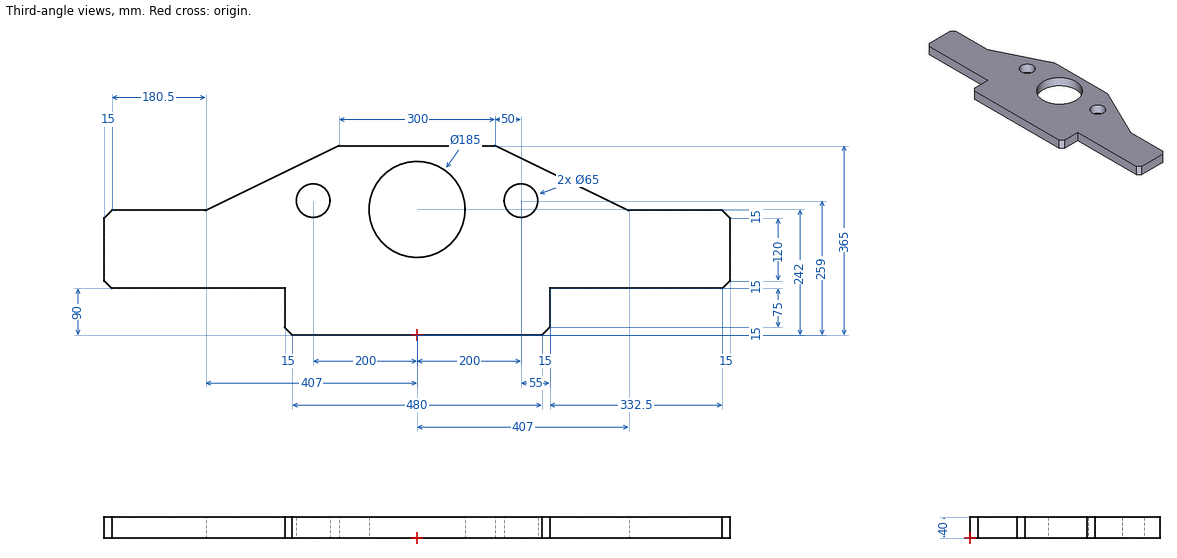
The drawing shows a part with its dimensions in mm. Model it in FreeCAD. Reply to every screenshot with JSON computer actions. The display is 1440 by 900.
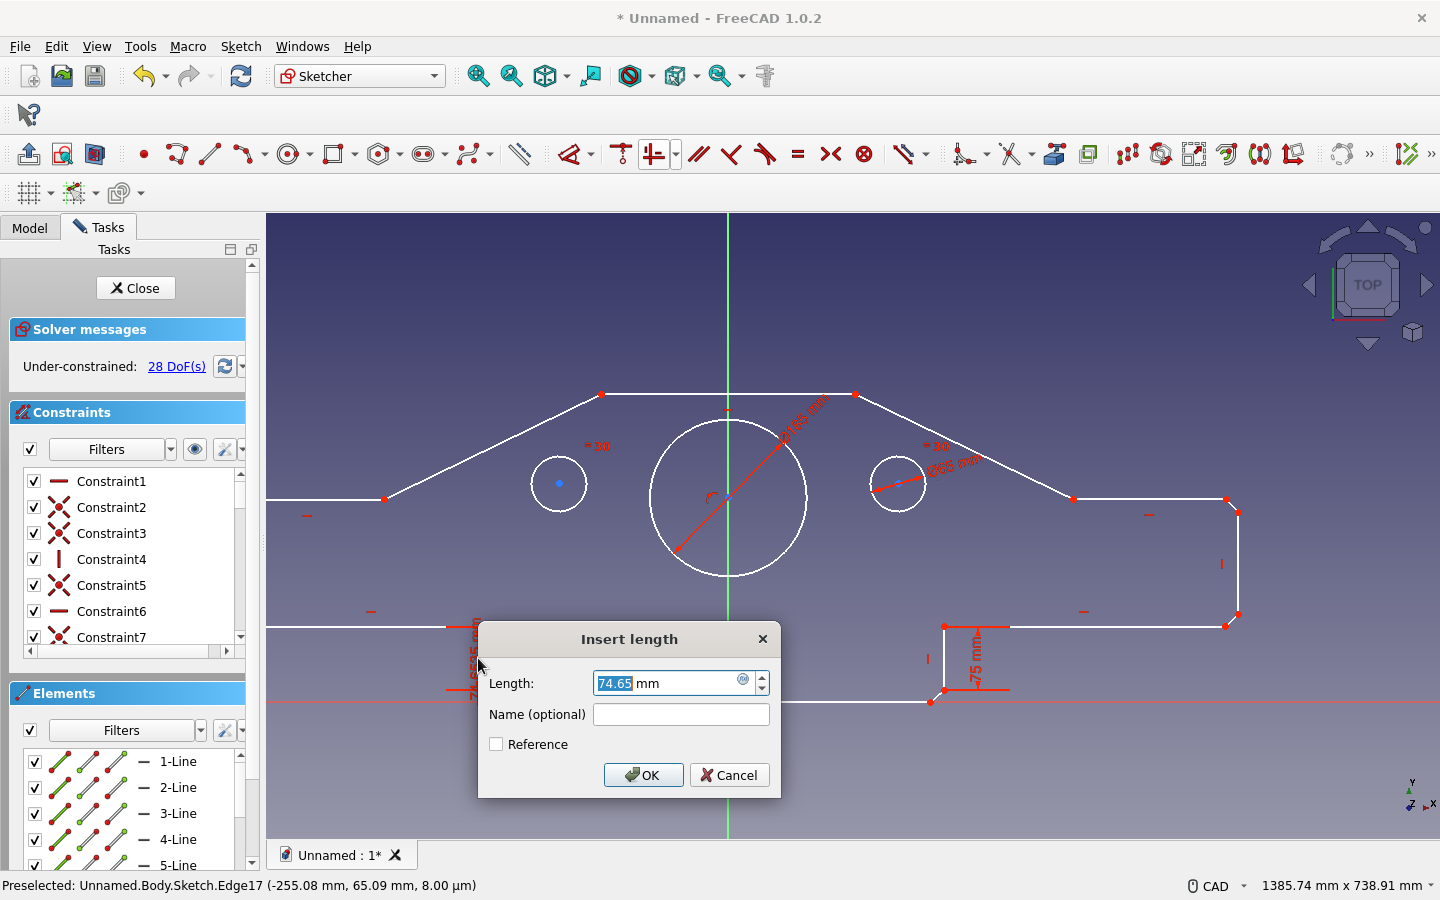
{"action": "type", "text": "75"}
{"action": "key", "text": "Return"}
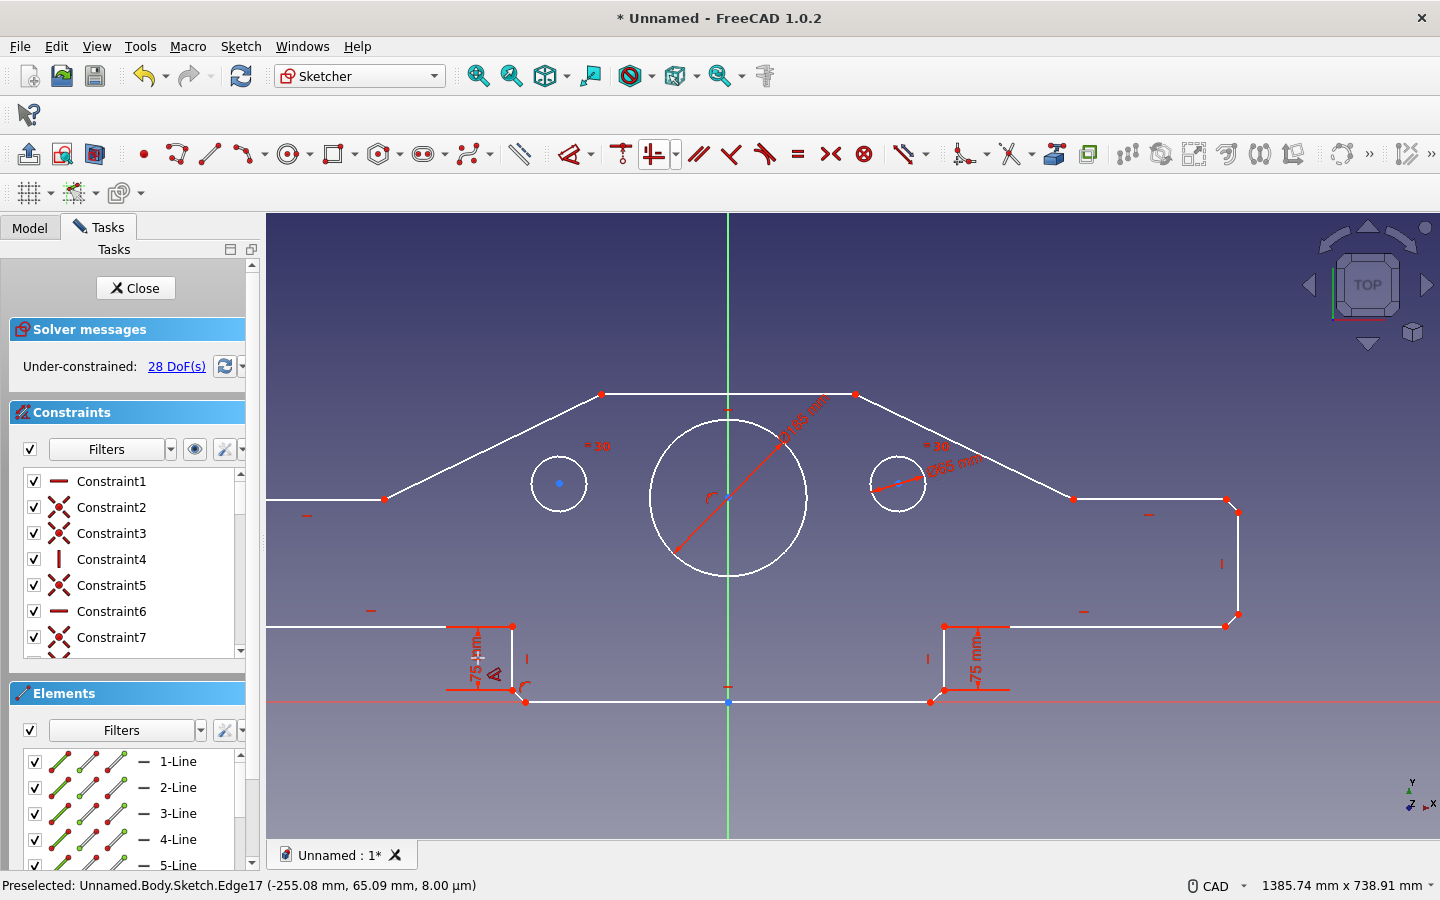
{"action": "left_click", "coordinate": [647, 702]}
{"action": "left_click", "coordinate": [635, 736]}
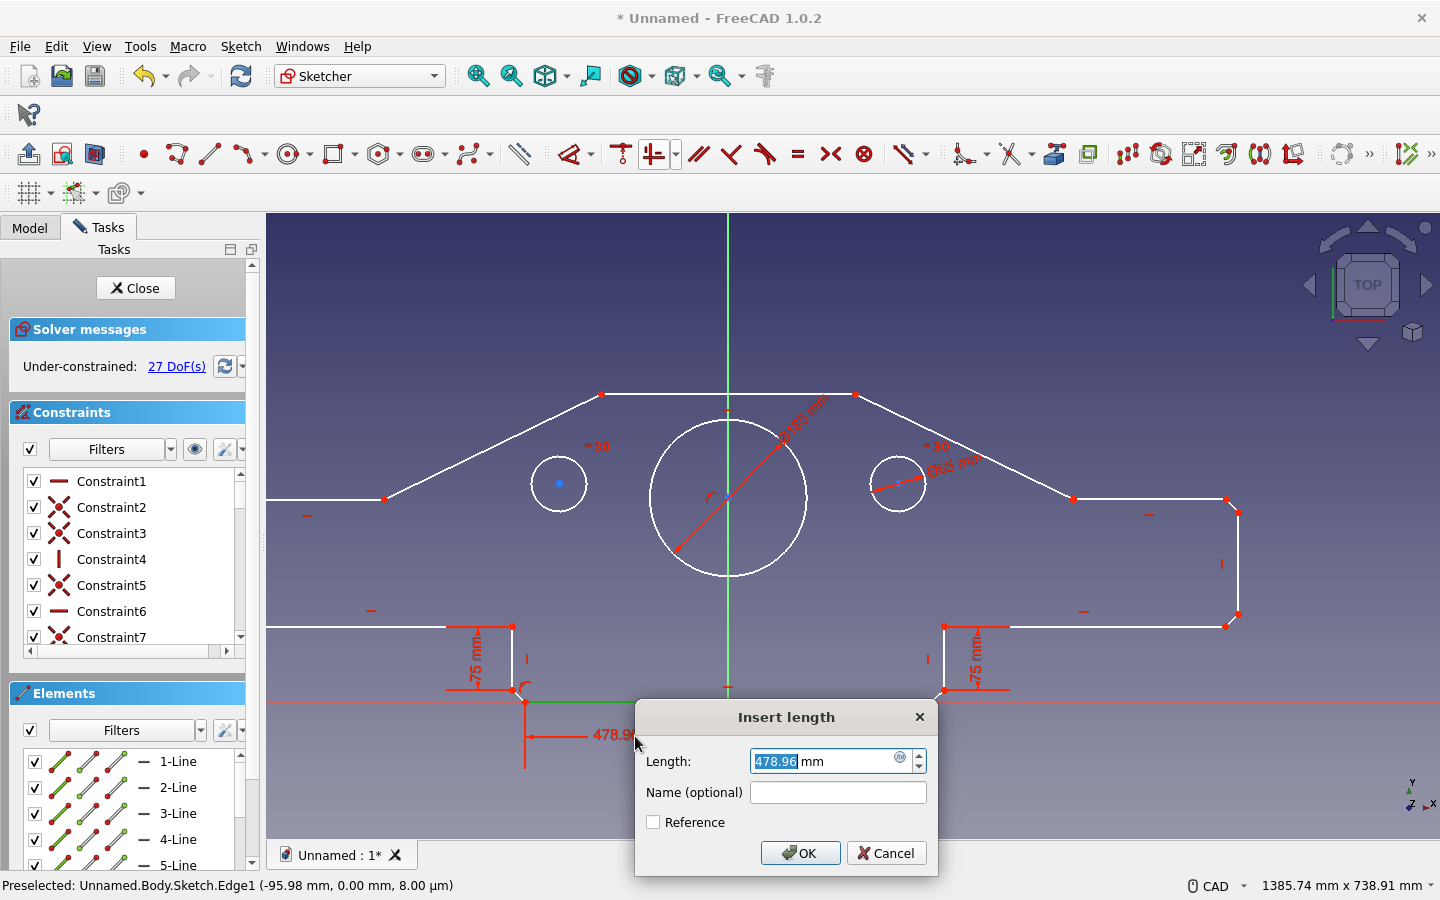
{"action": "type", "text": "480"}
{"action": "key", "text": "Return"}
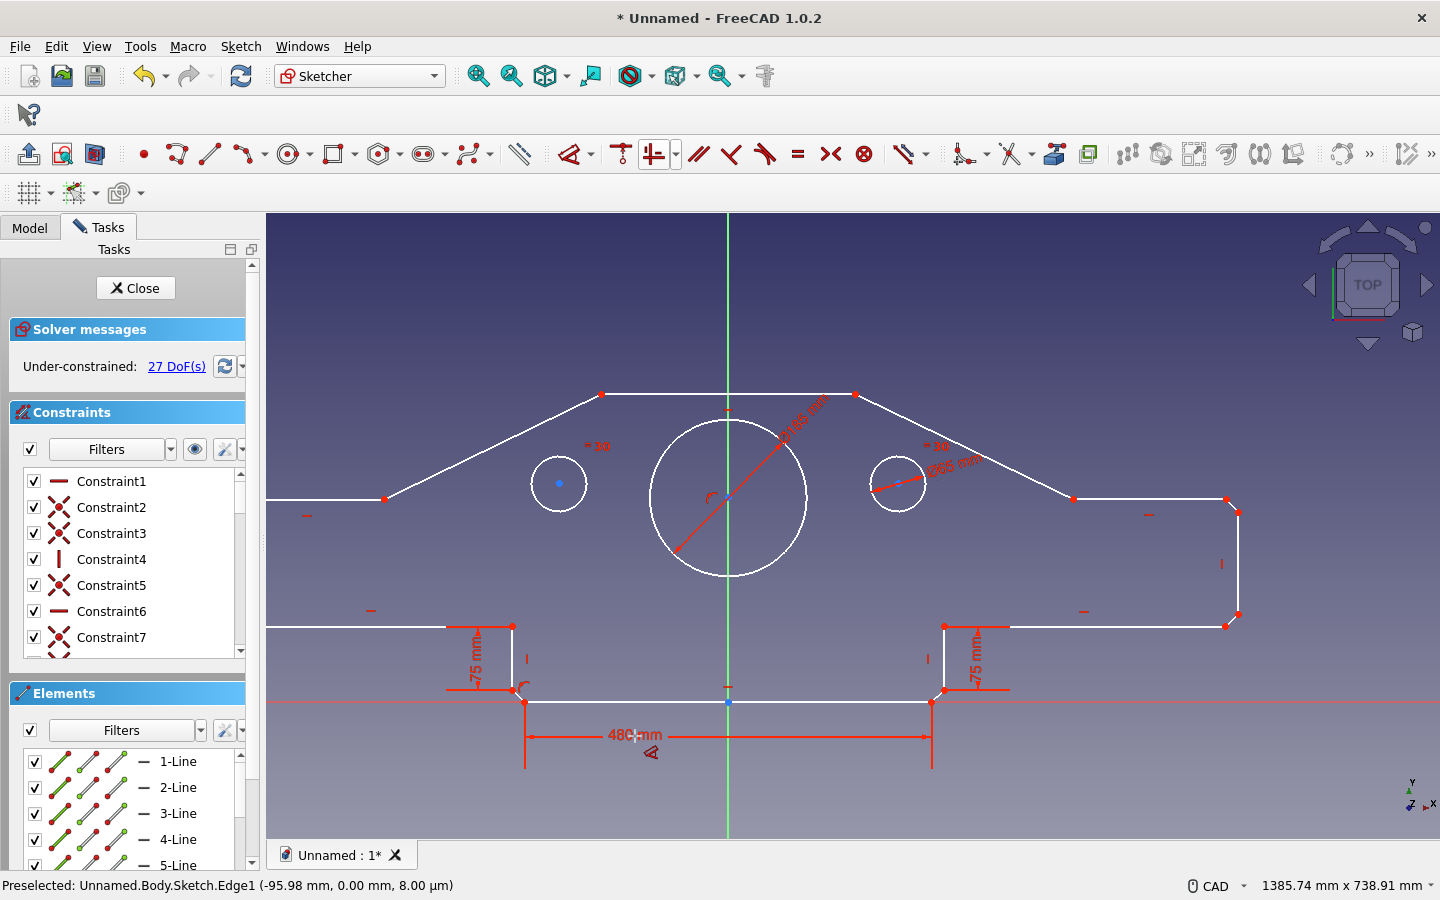
{"action": "left_click", "coordinate": [1238, 584]}
{"action": "left_click", "coordinate": [1272, 563]}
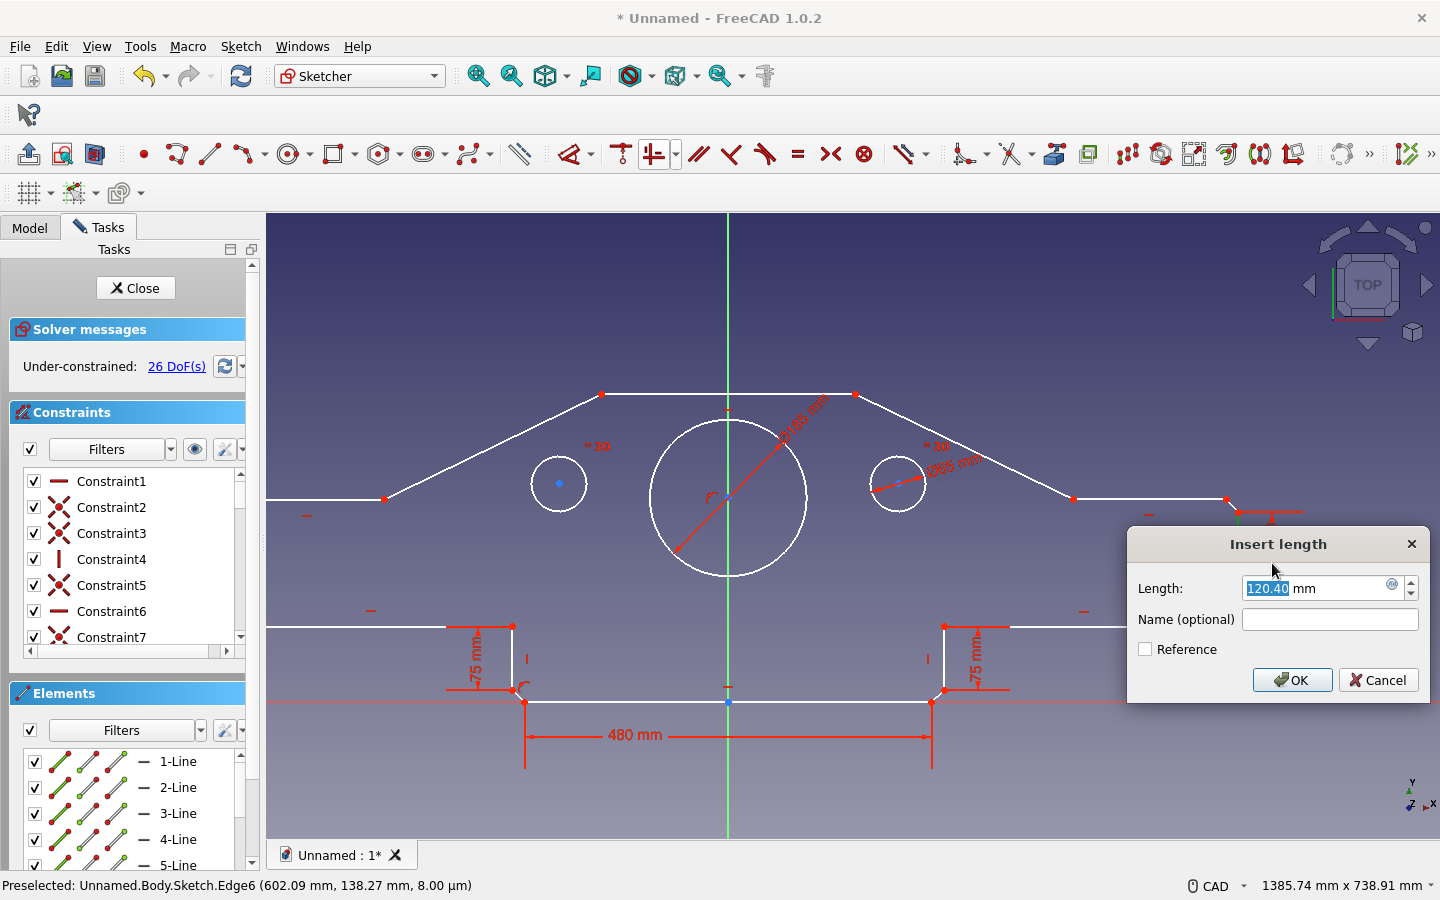
{"action": "type", "text": "120"}
{"action": "key", "text": "Return"}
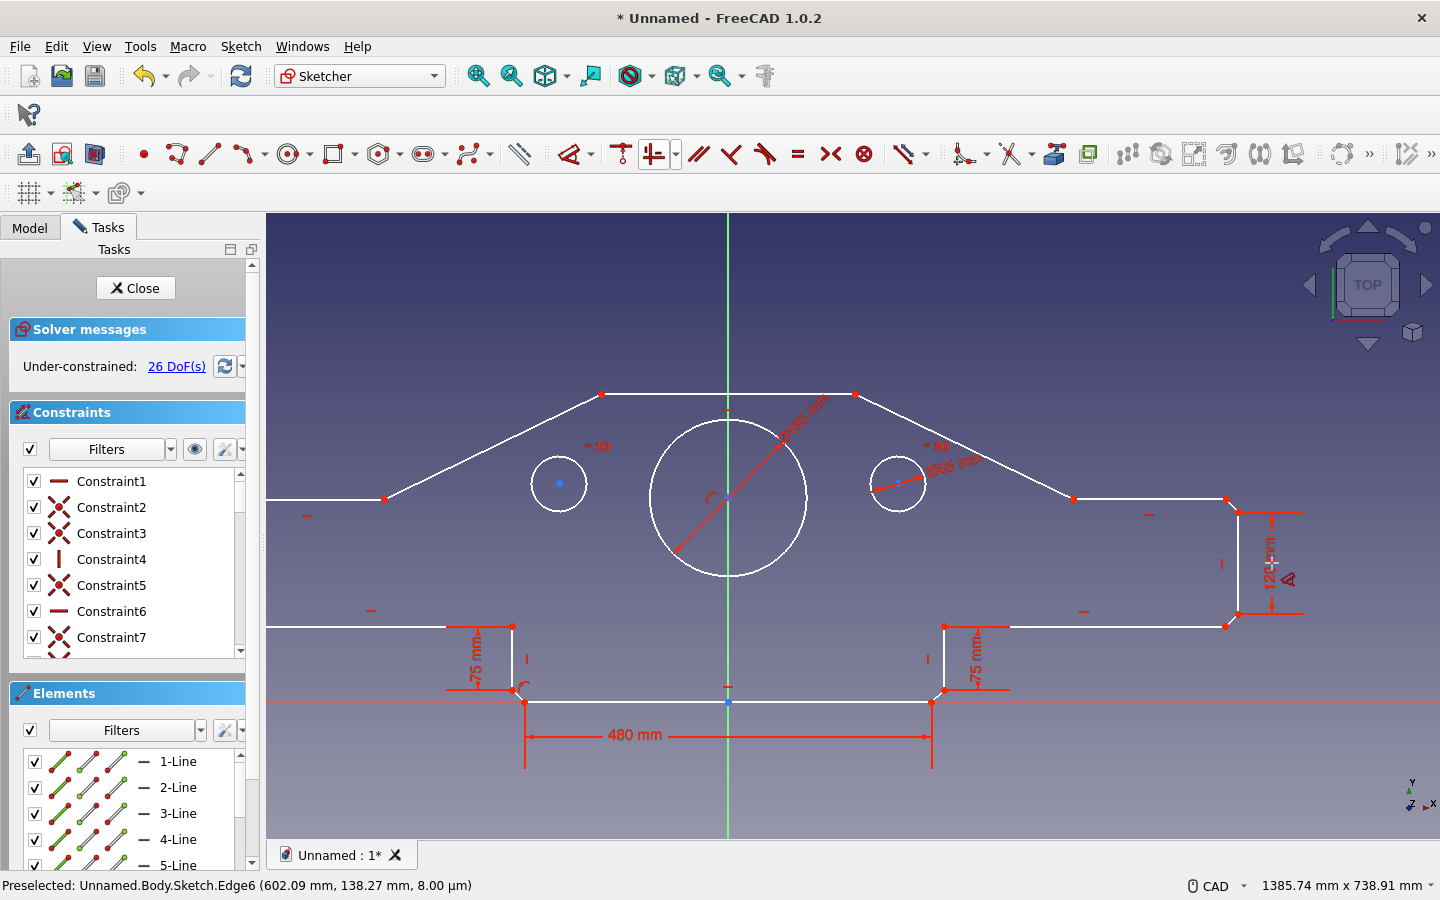
{"action": "left_click", "coordinate": [779, 394]}
{"action": "left_click", "coordinate": [670, 360]}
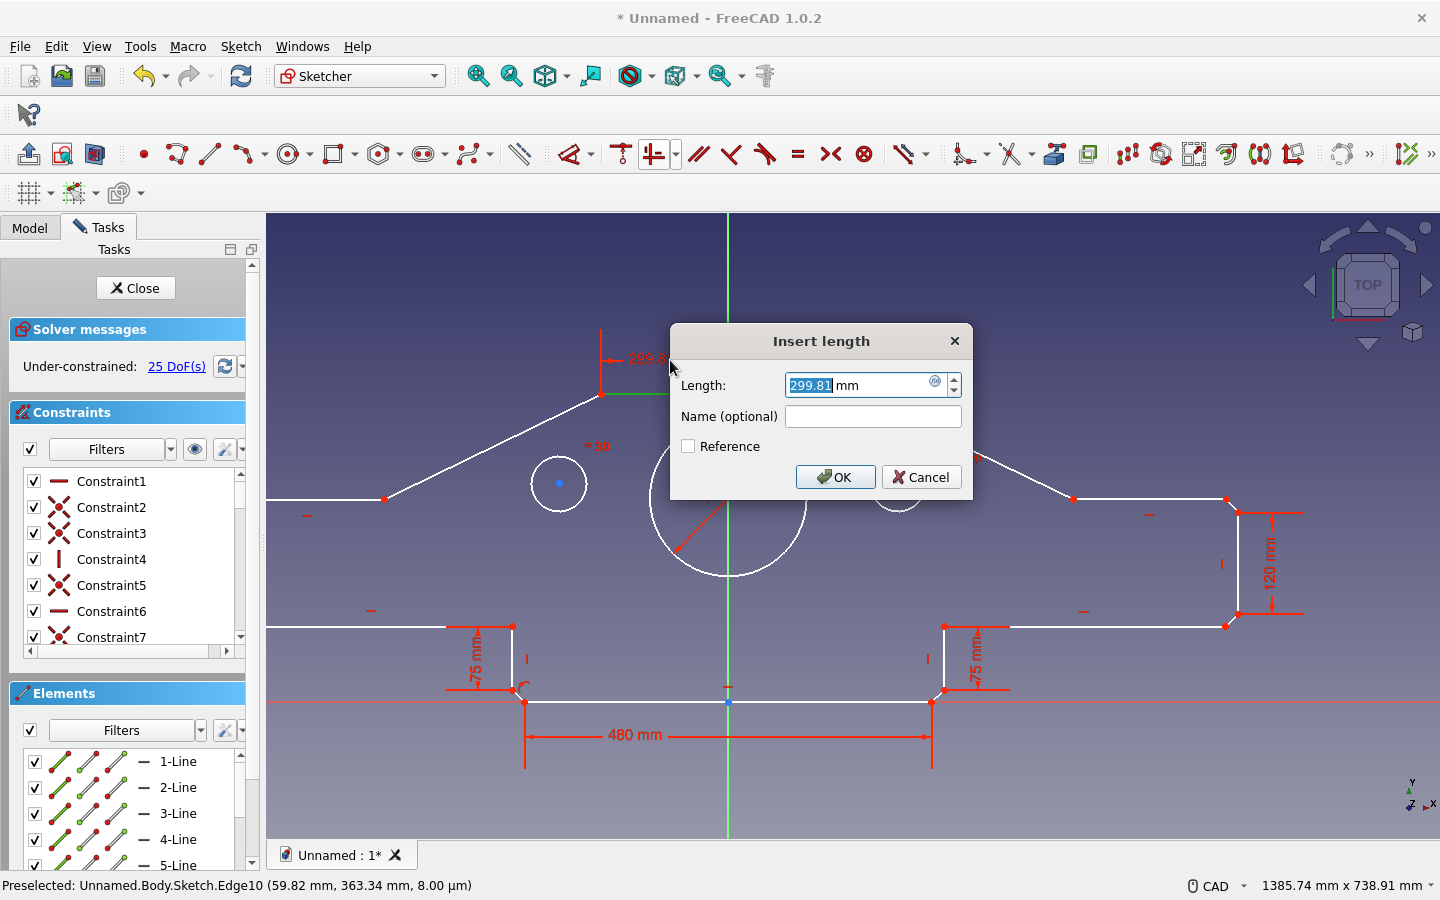
{"action": "type", "text": "300"}
{"action": "key", "text": "Return"}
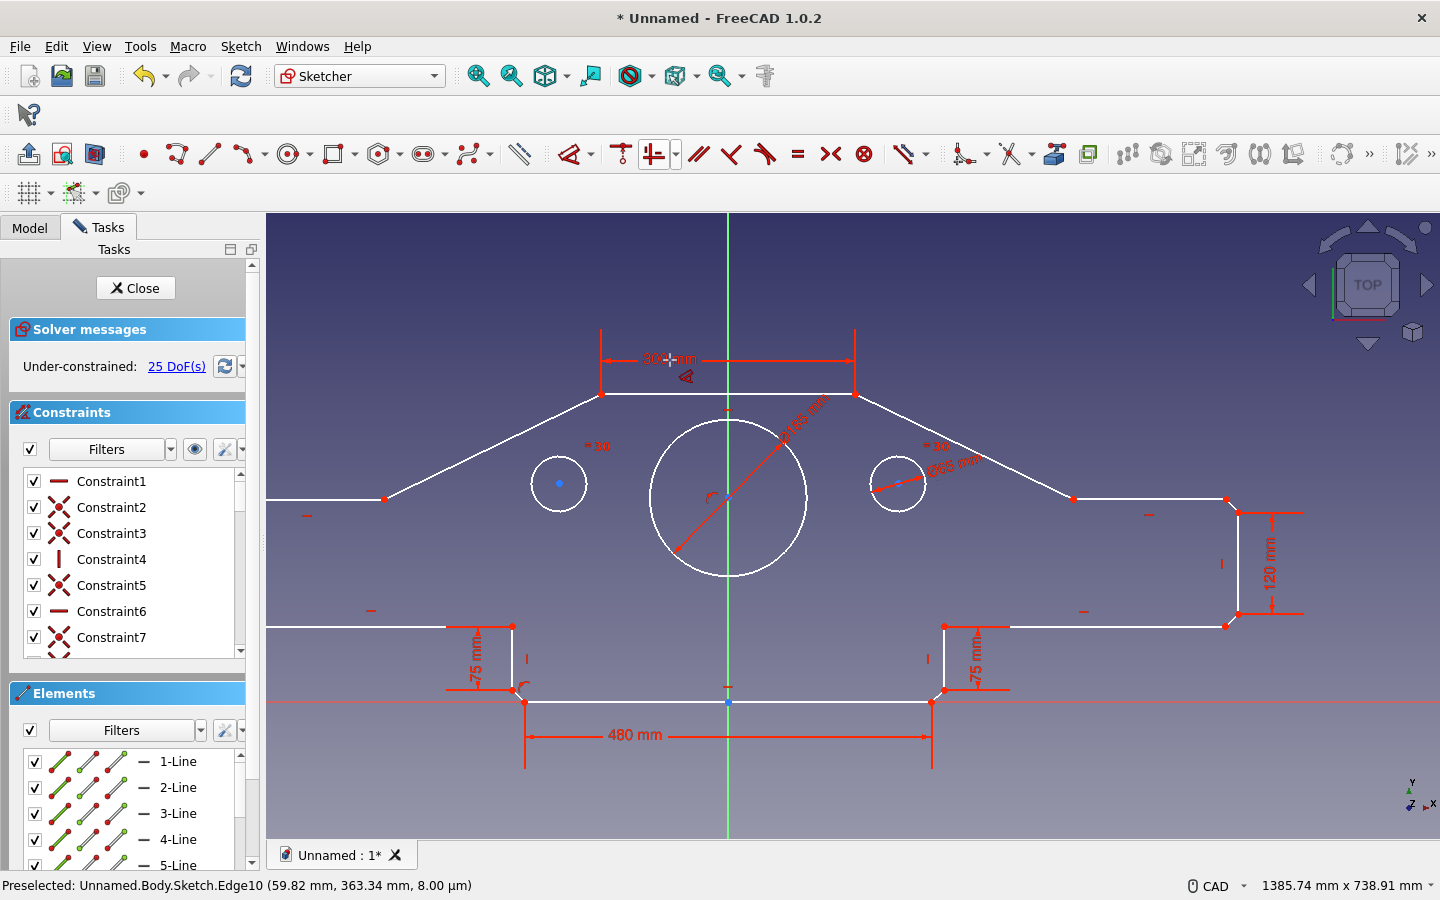
{"action": "scroll", "coordinate": [899, 482], "scroll_direction": "down", "scroll_amount": 2}